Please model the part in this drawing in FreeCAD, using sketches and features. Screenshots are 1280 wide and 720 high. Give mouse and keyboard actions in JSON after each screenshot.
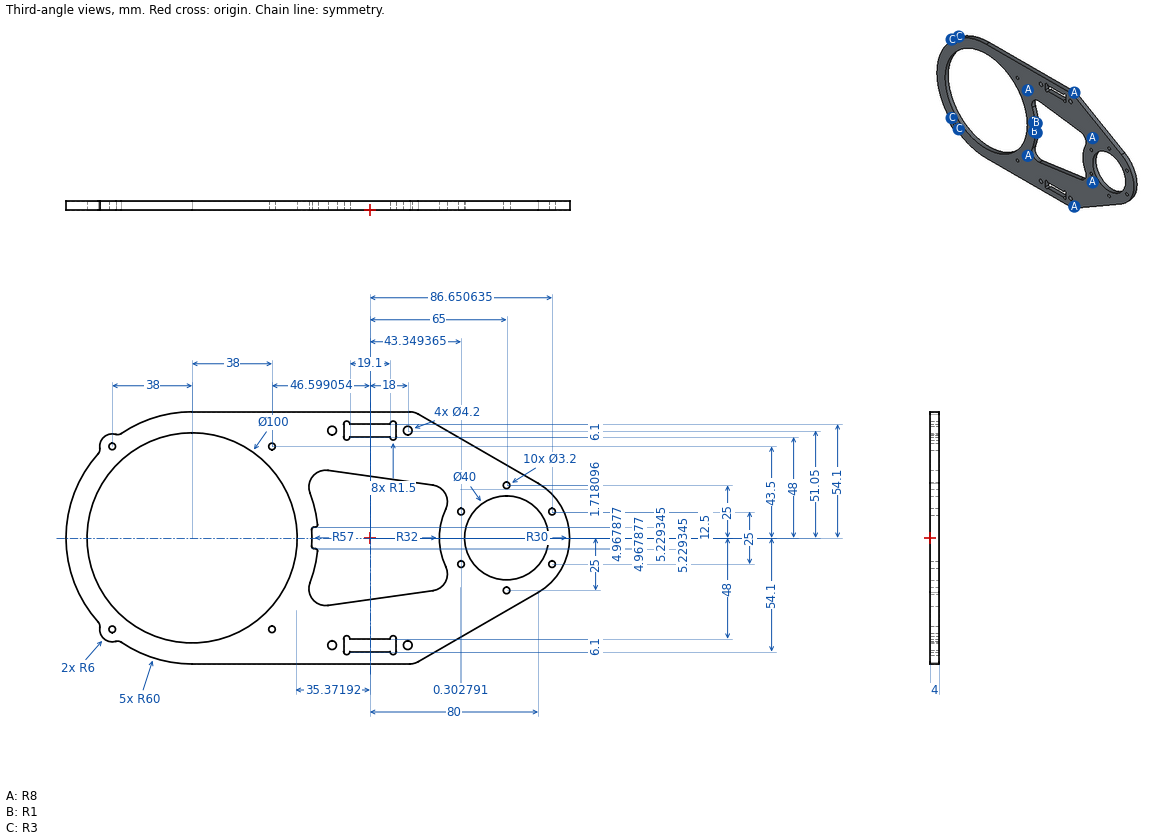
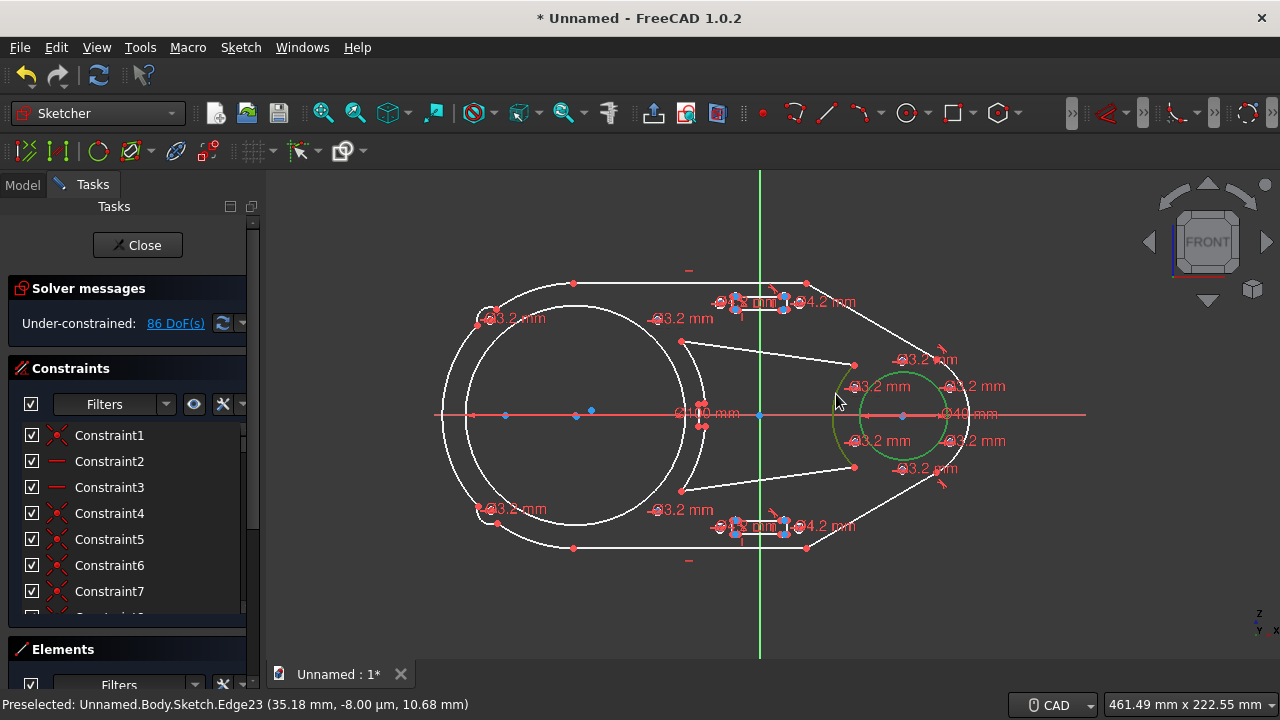
{"action": "key", "text": "c"}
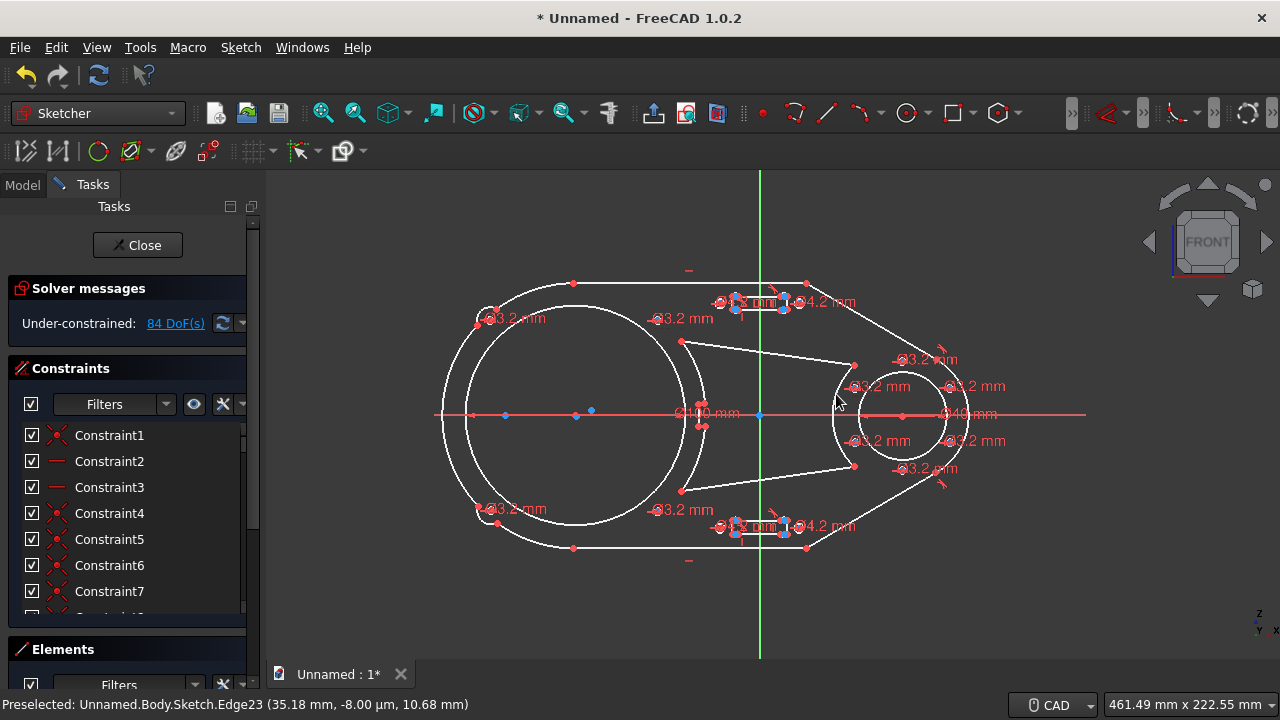
{"action": "left_click", "coordinate": [653, 337]}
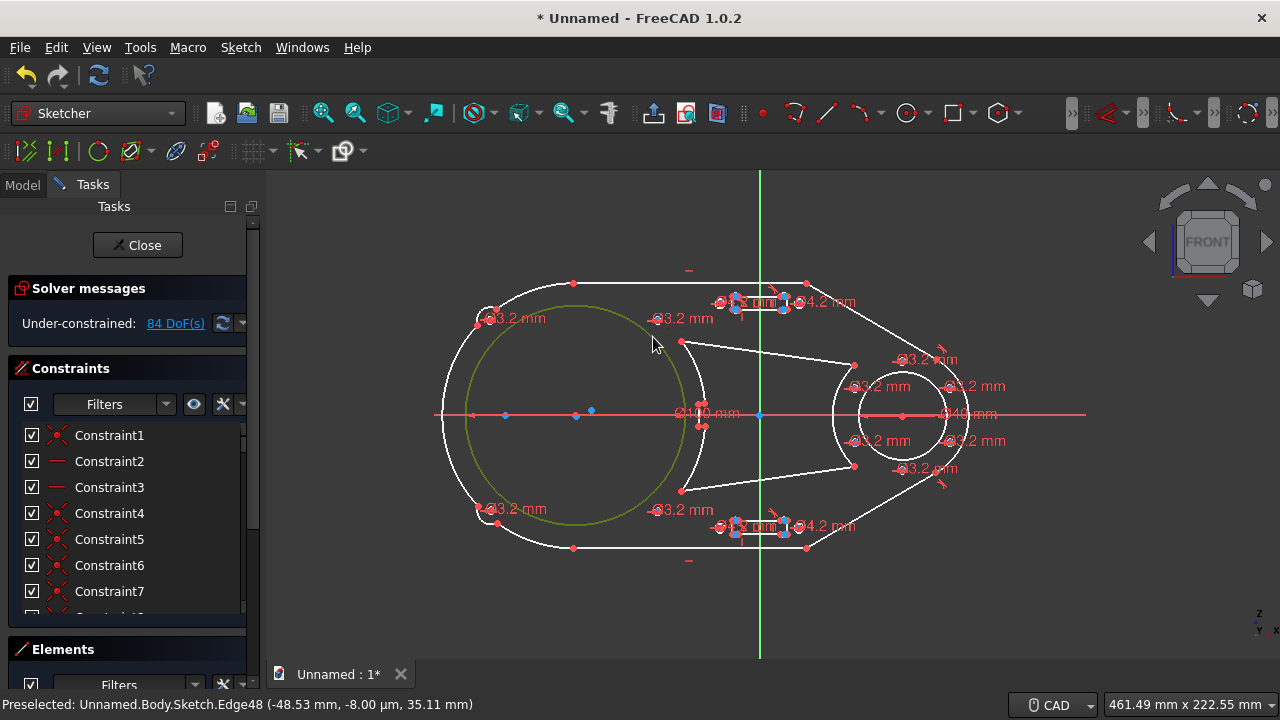
{"action": "left_click", "coordinate": [702, 384]}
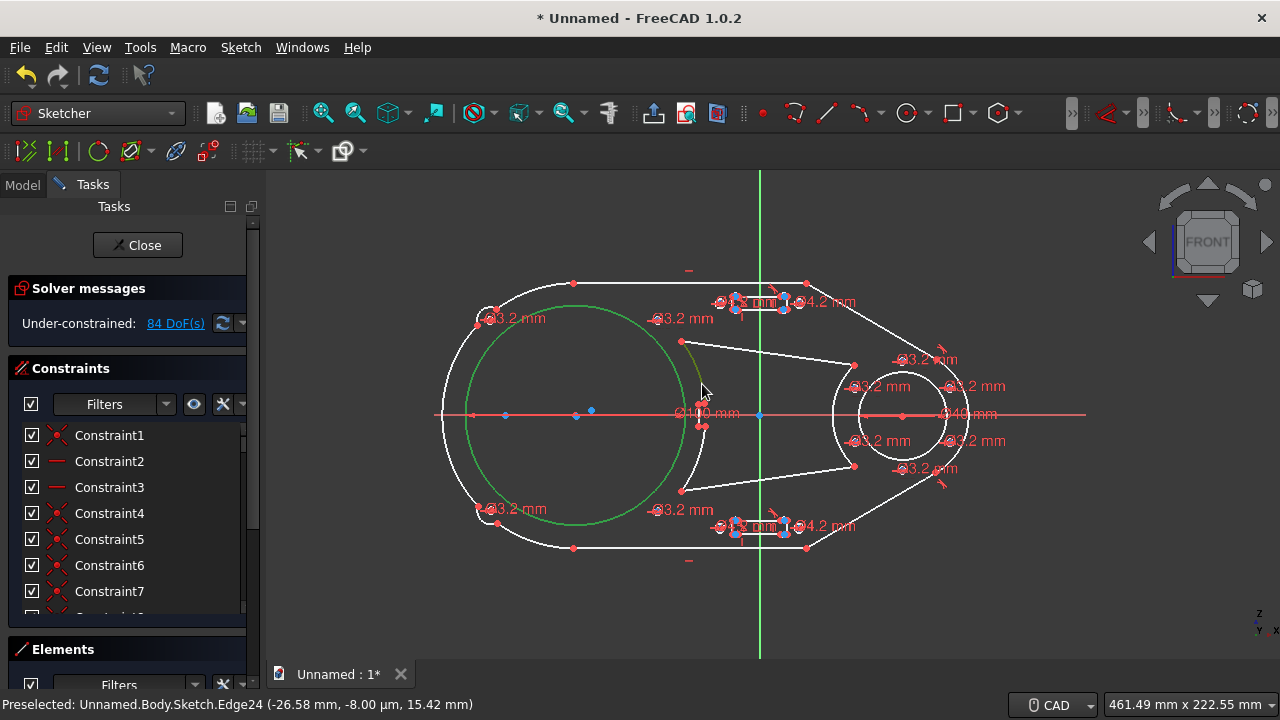
{"action": "key", "text": "c"}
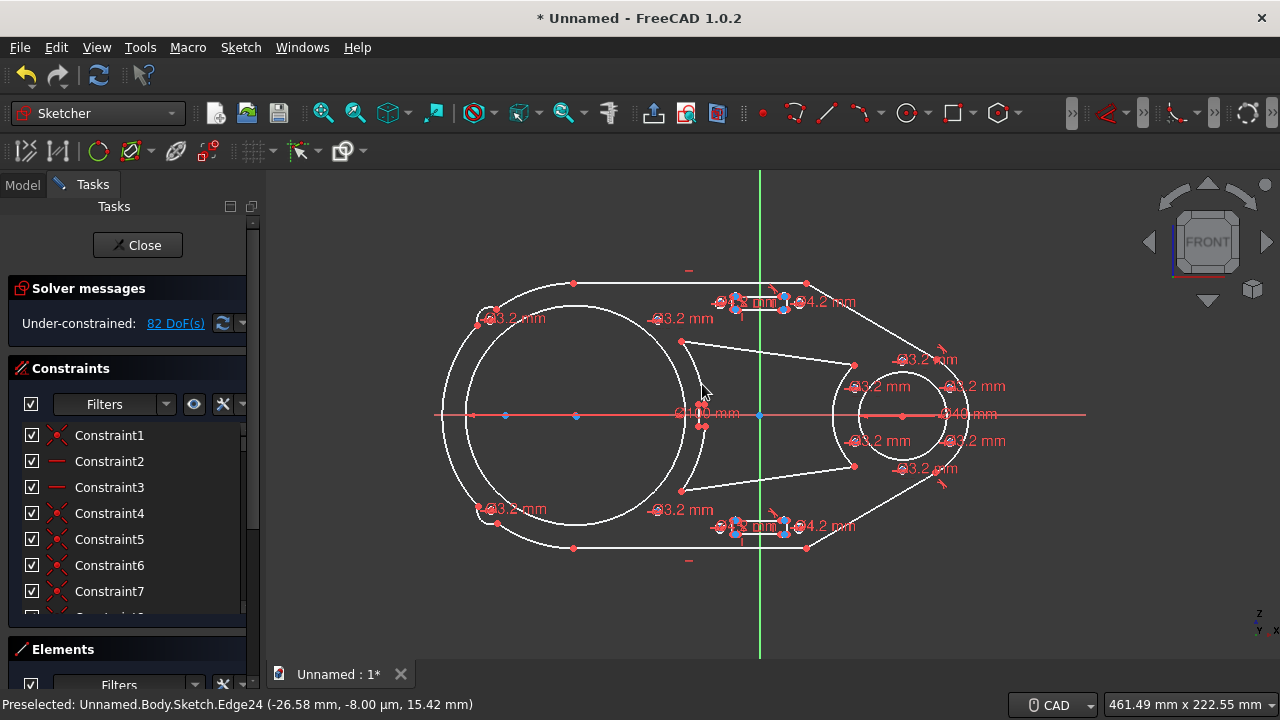
{"action": "left_click", "coordinate": [653, 337]}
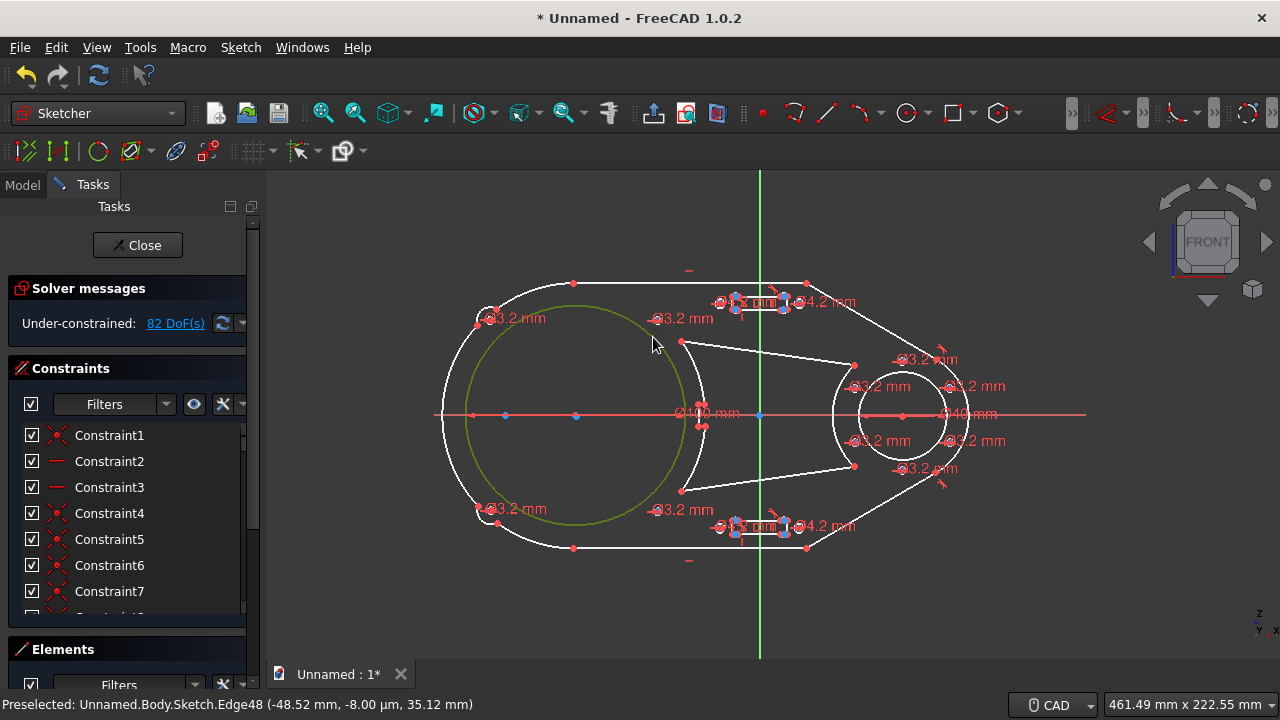
{"action": "scroll", "coordinate": [699, 415], "scroll_direction": "up", "scroll_amount": 2}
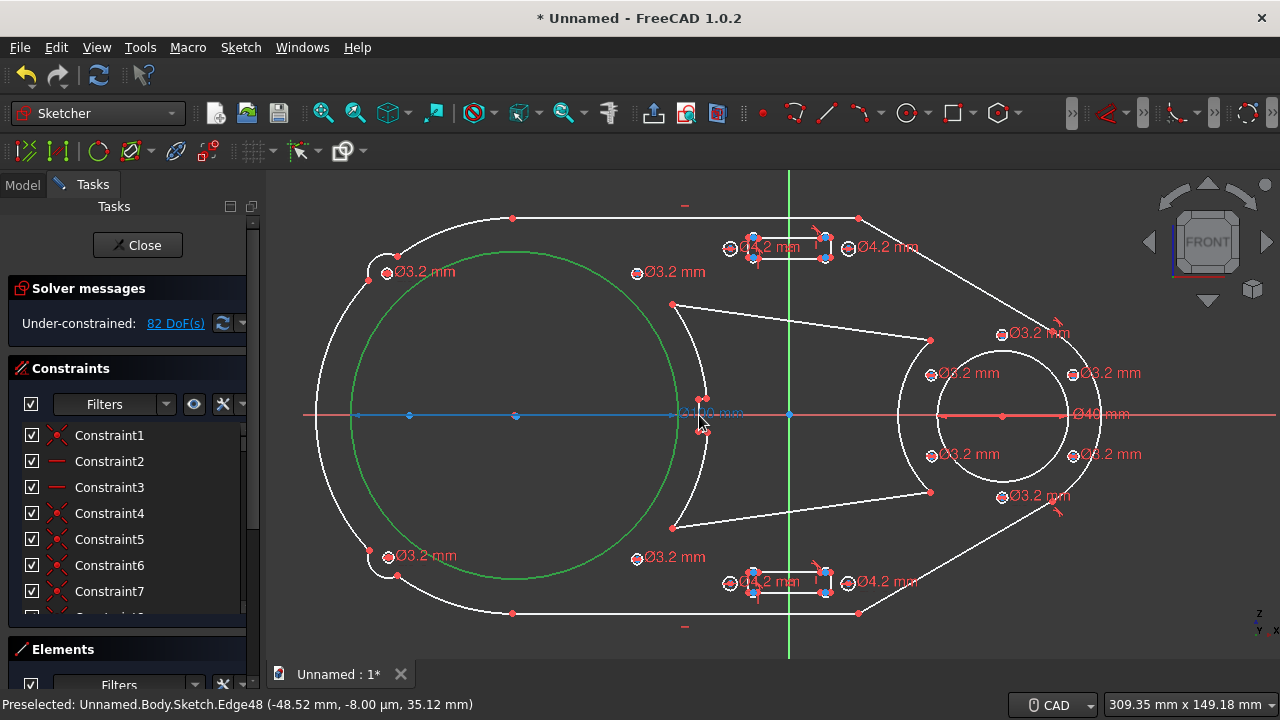
{"action": "left_click", "coordinate": [699, 422]}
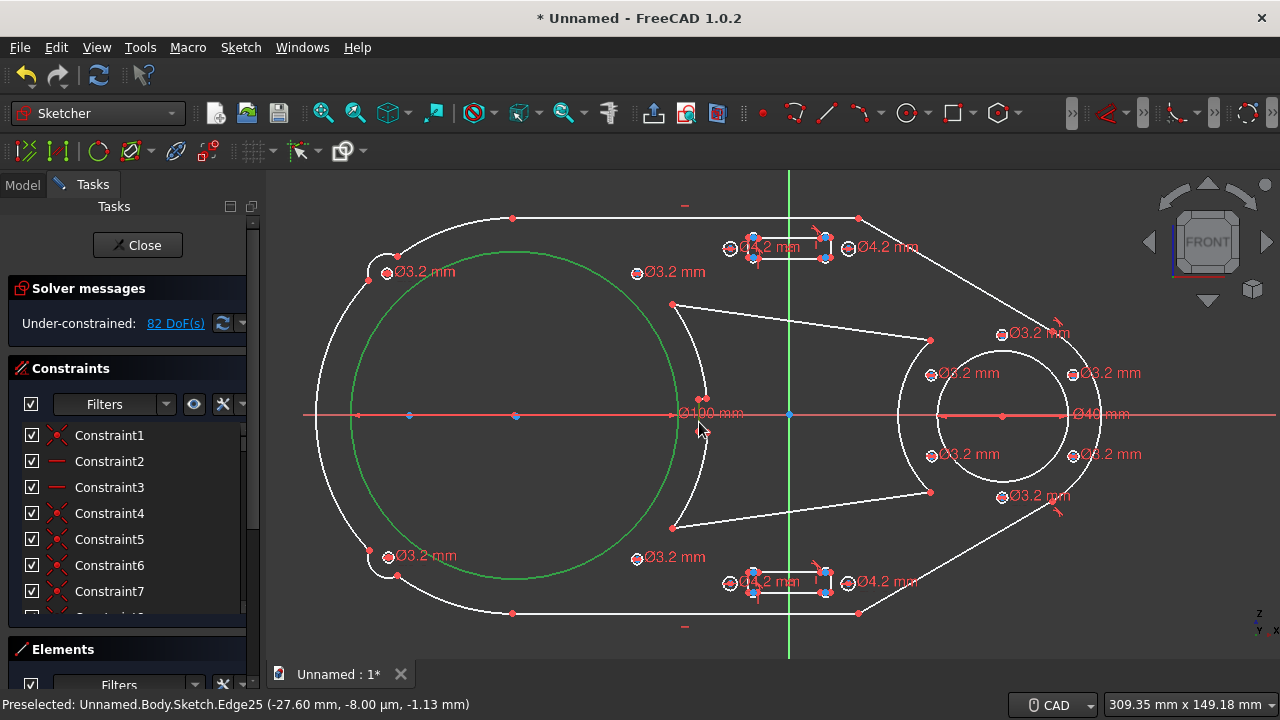
{"action": "key", "text": "c"}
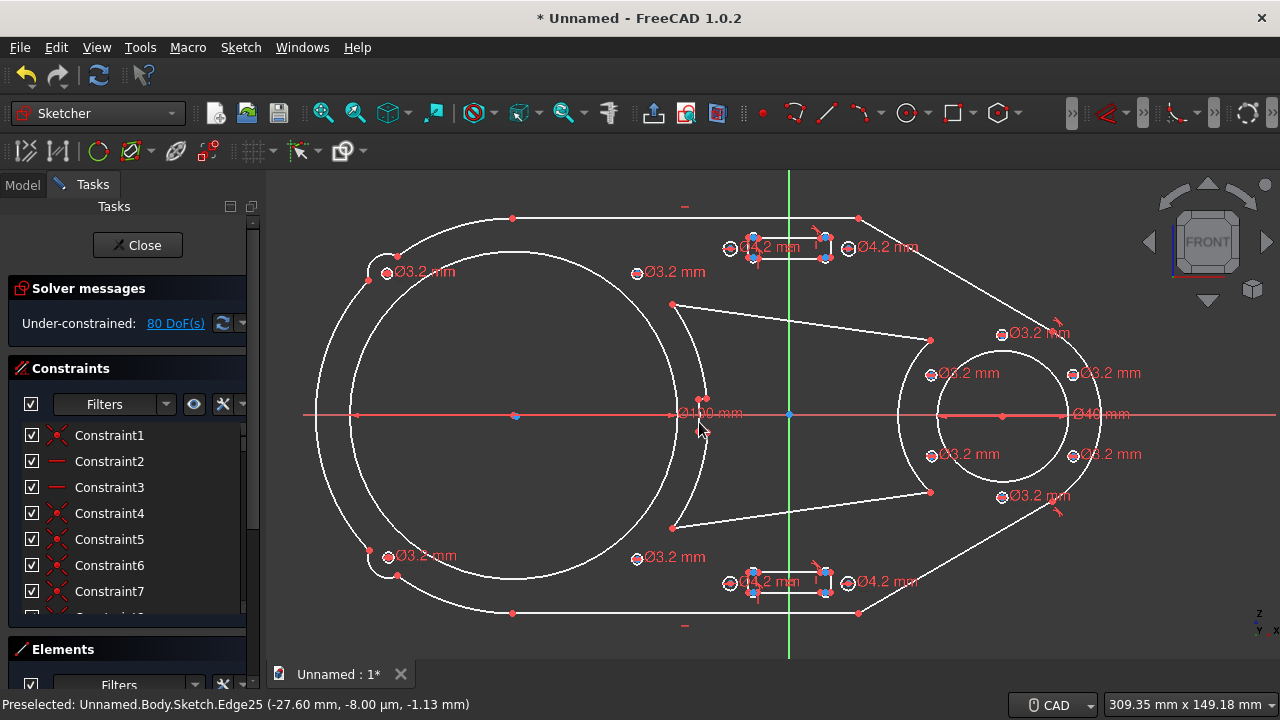
{"action": "left_click", "coordinate": [629, 299]}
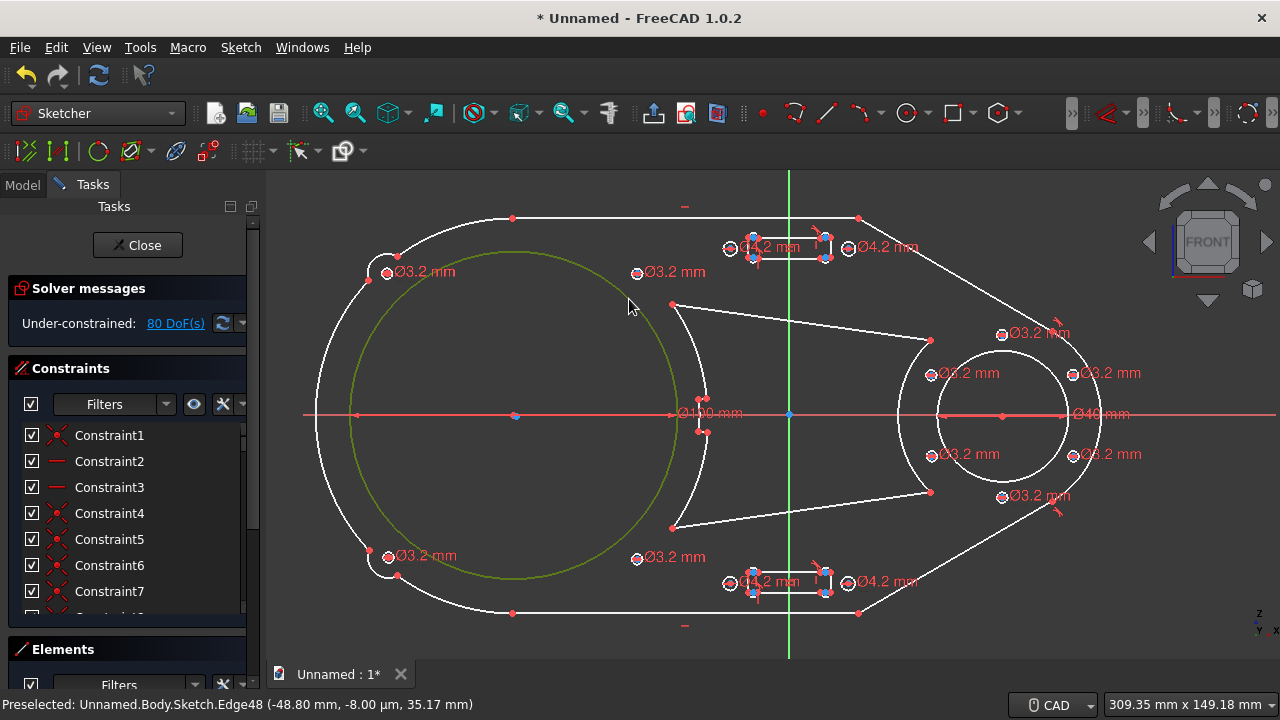
{"action": "left_click", "coordinate": [689, 502]}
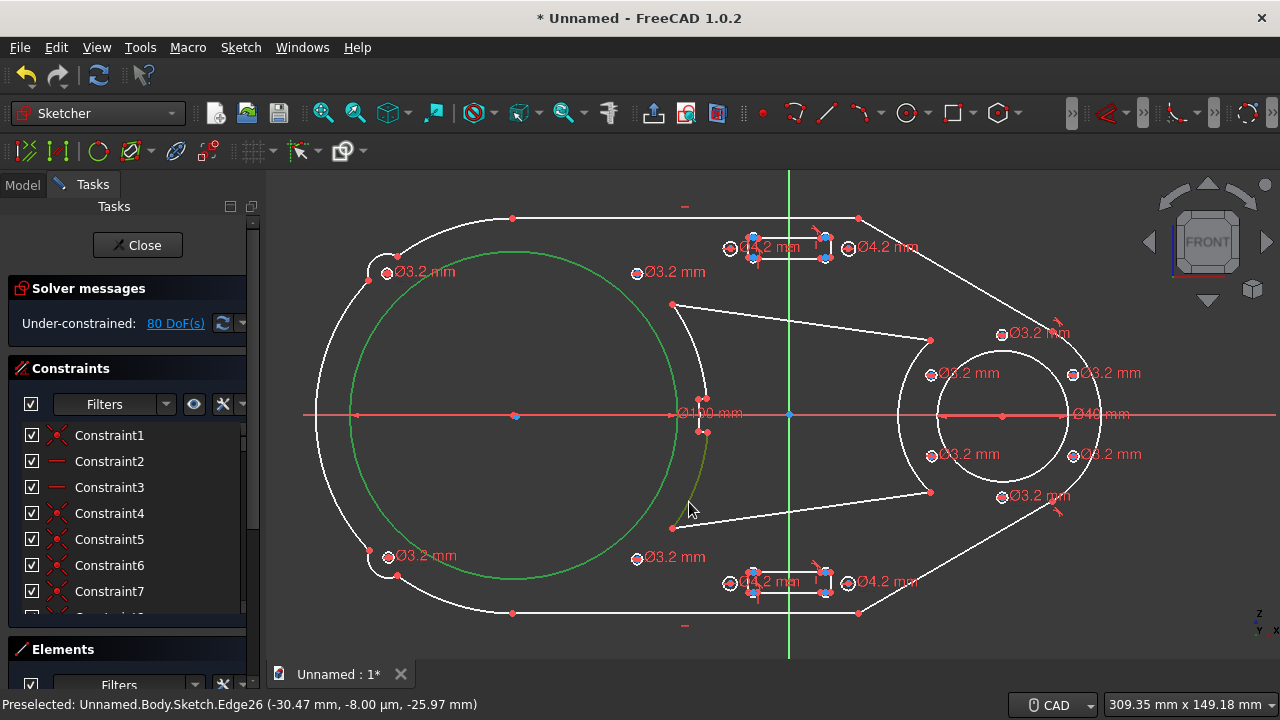
{"action": "key", "text": "c"}